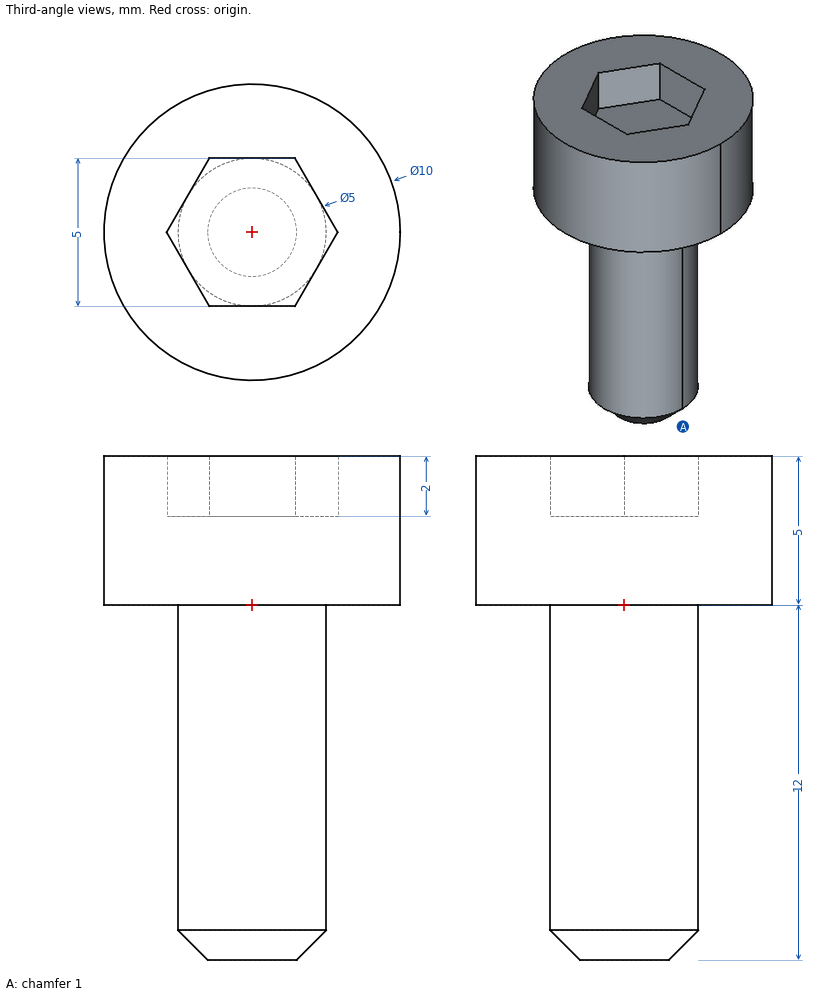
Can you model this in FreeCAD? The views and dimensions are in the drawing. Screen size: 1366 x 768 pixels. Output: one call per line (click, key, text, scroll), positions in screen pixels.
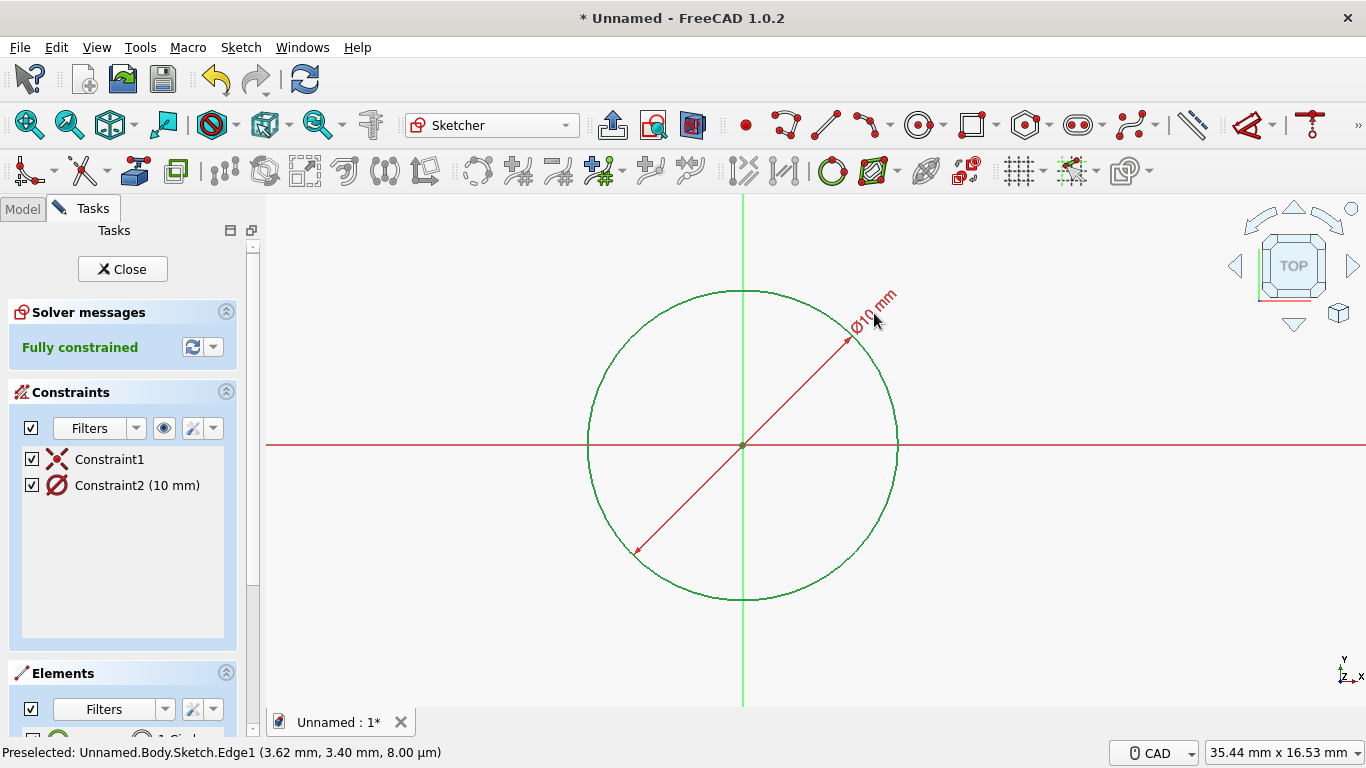
click(123, 269)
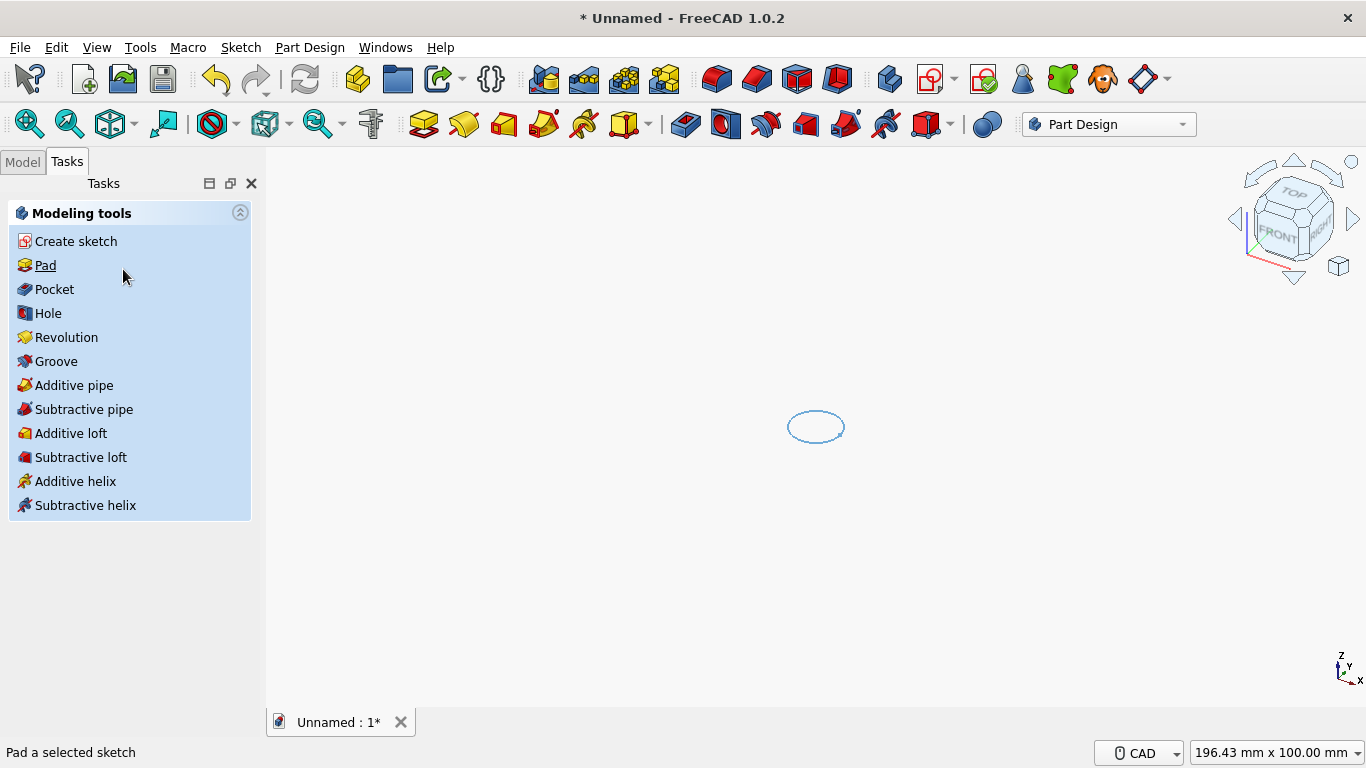
click(424, 124)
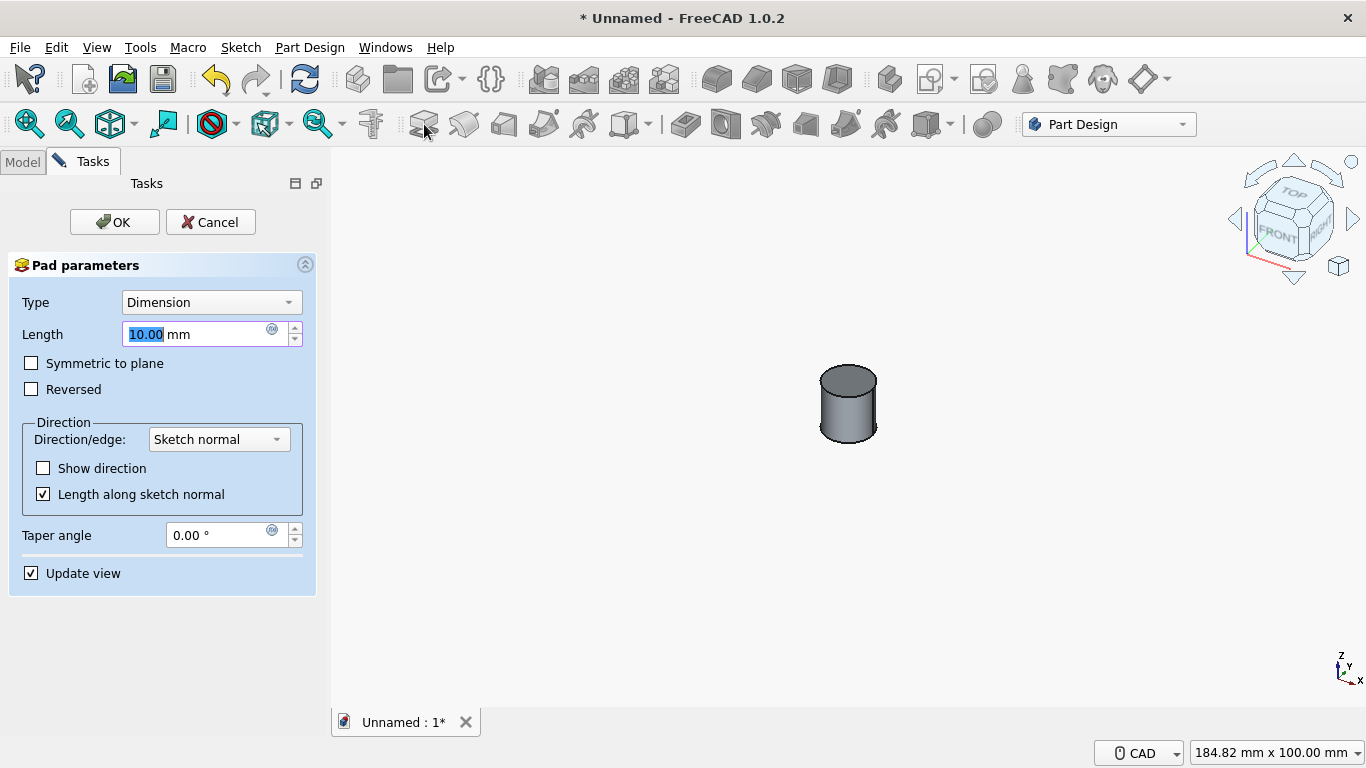
text(5)
key(Tab)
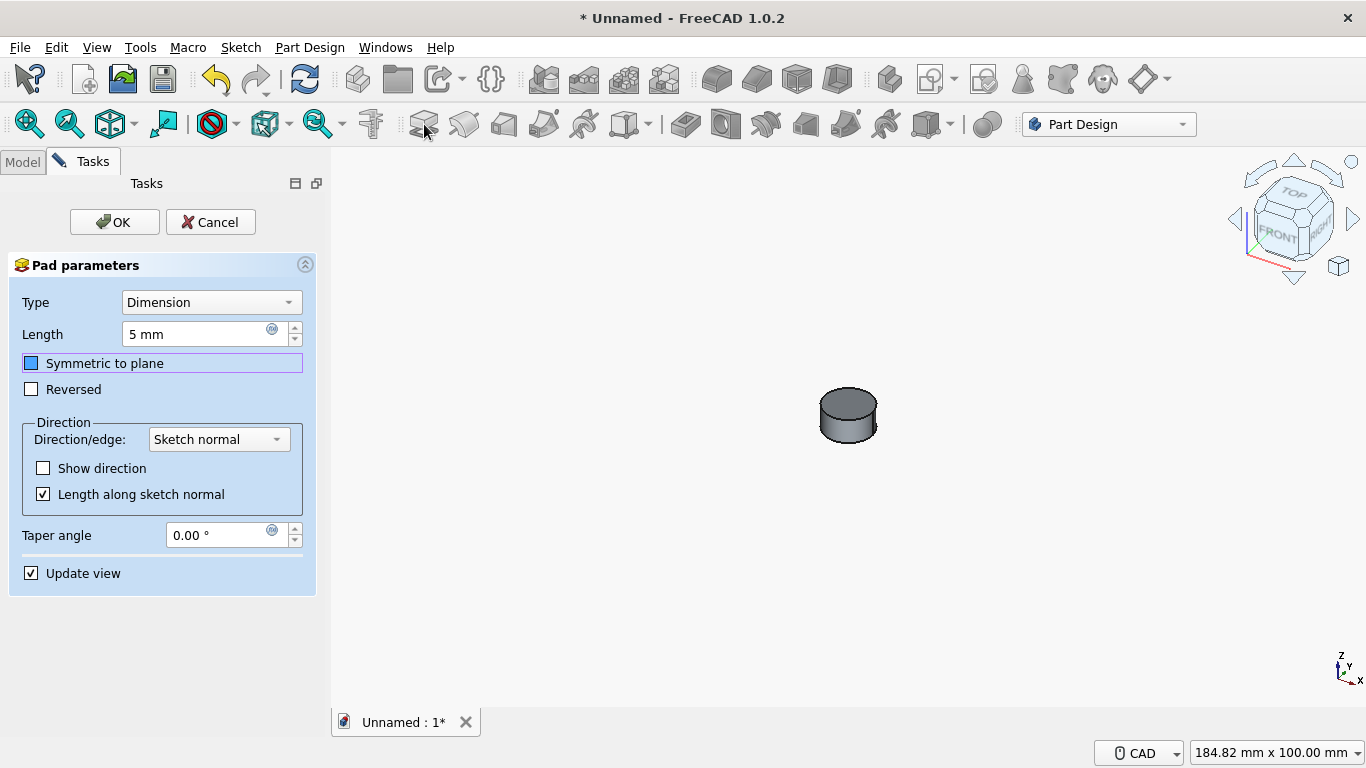
click(115, 222)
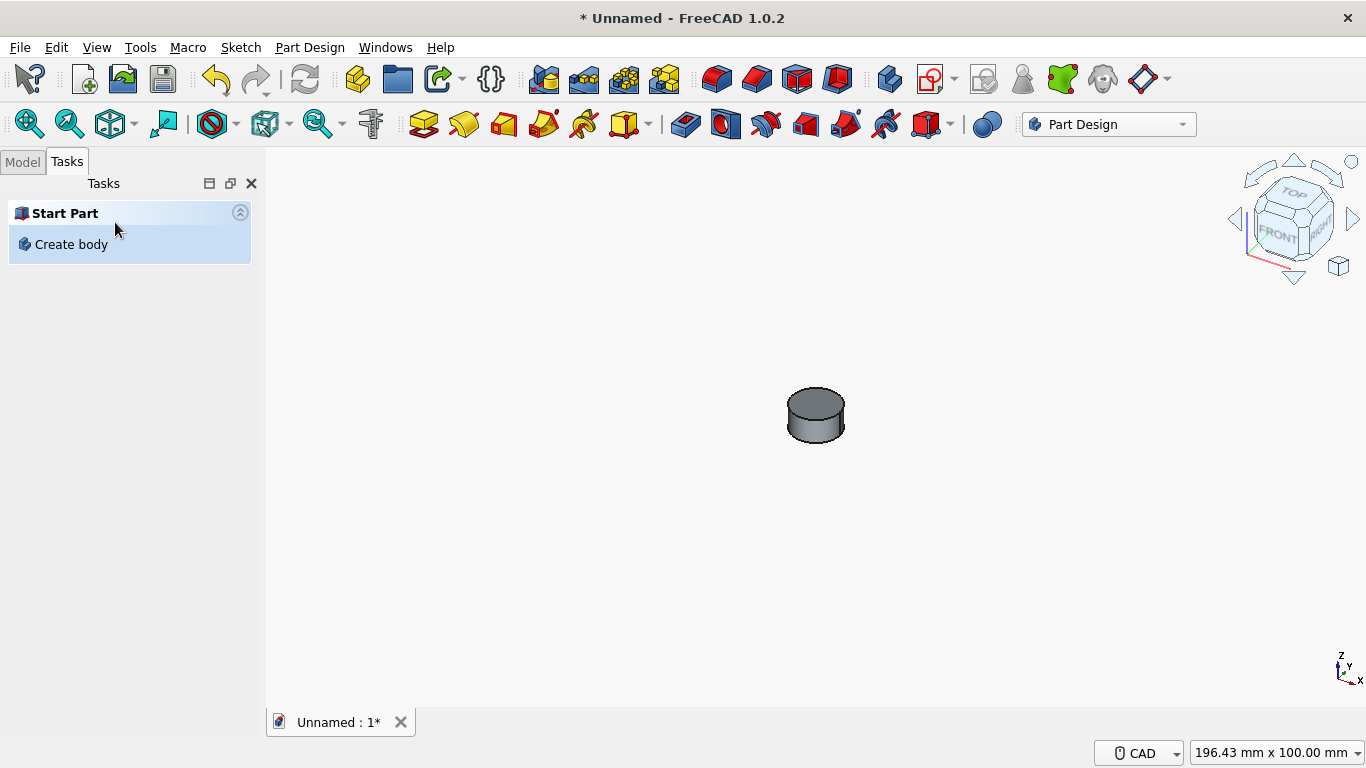
click(30, 124)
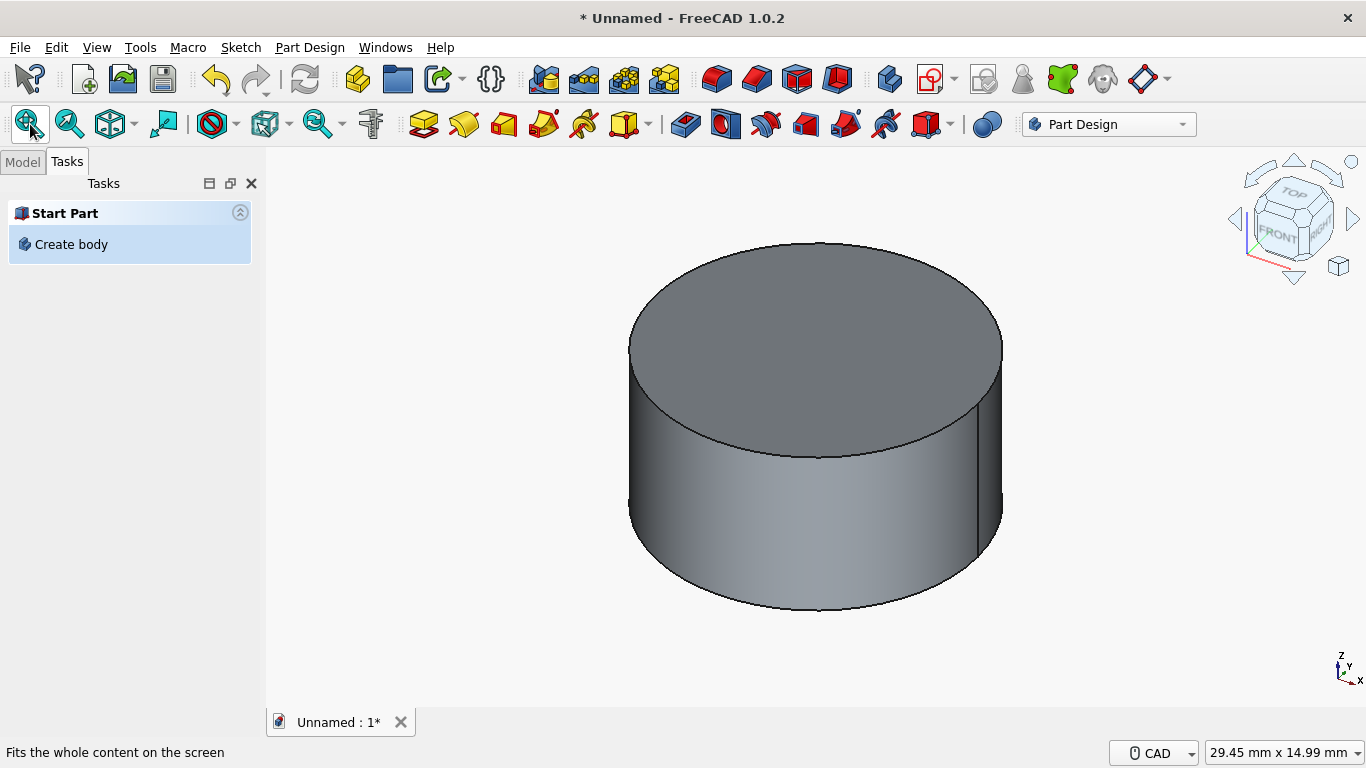
click(816, 349)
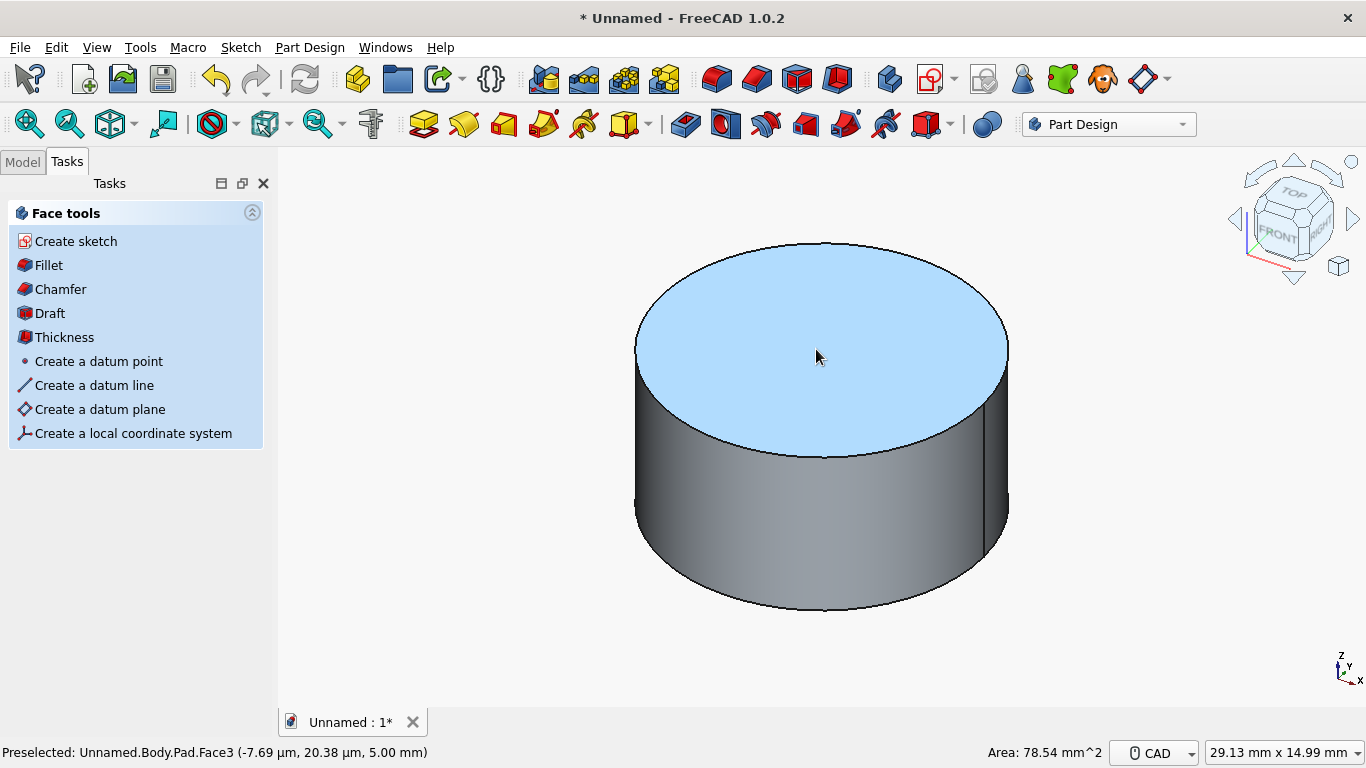
click(930, 80)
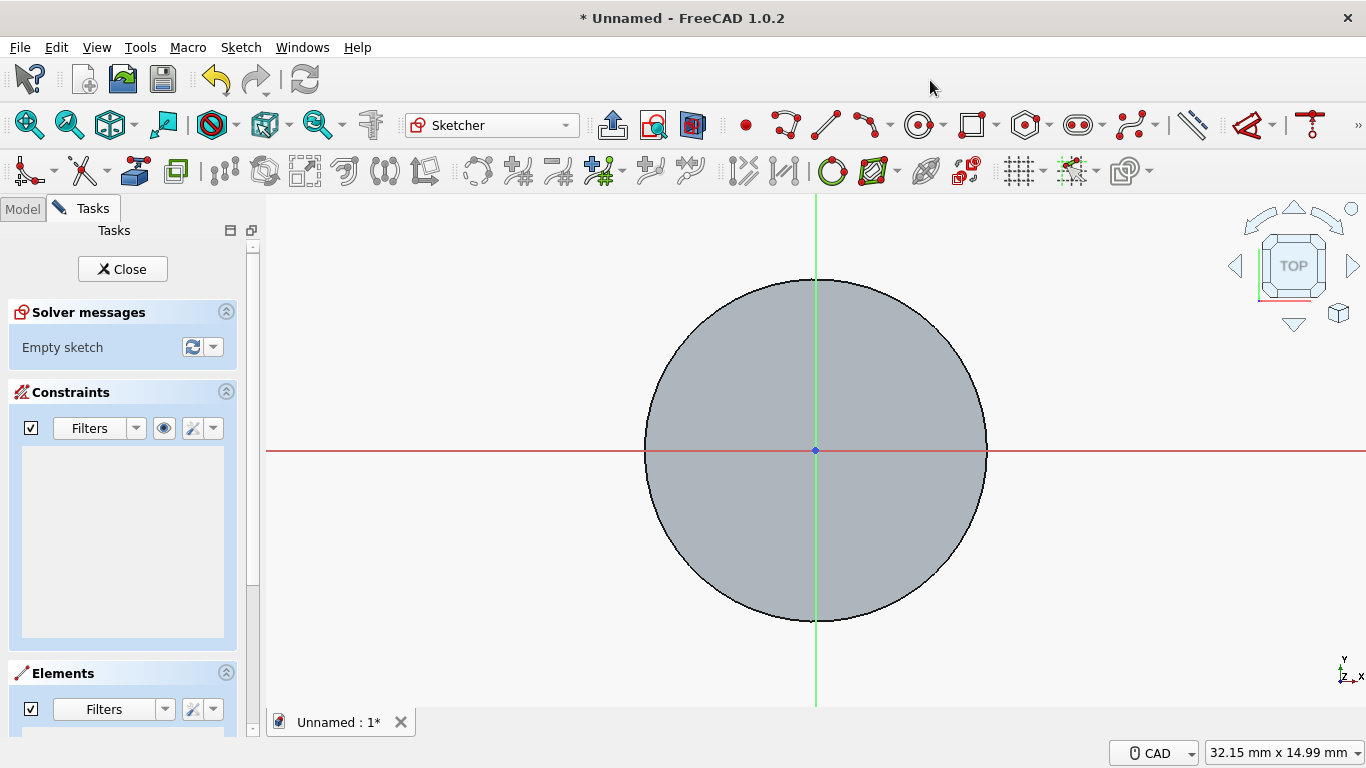
scroll(899, 450, up, 3)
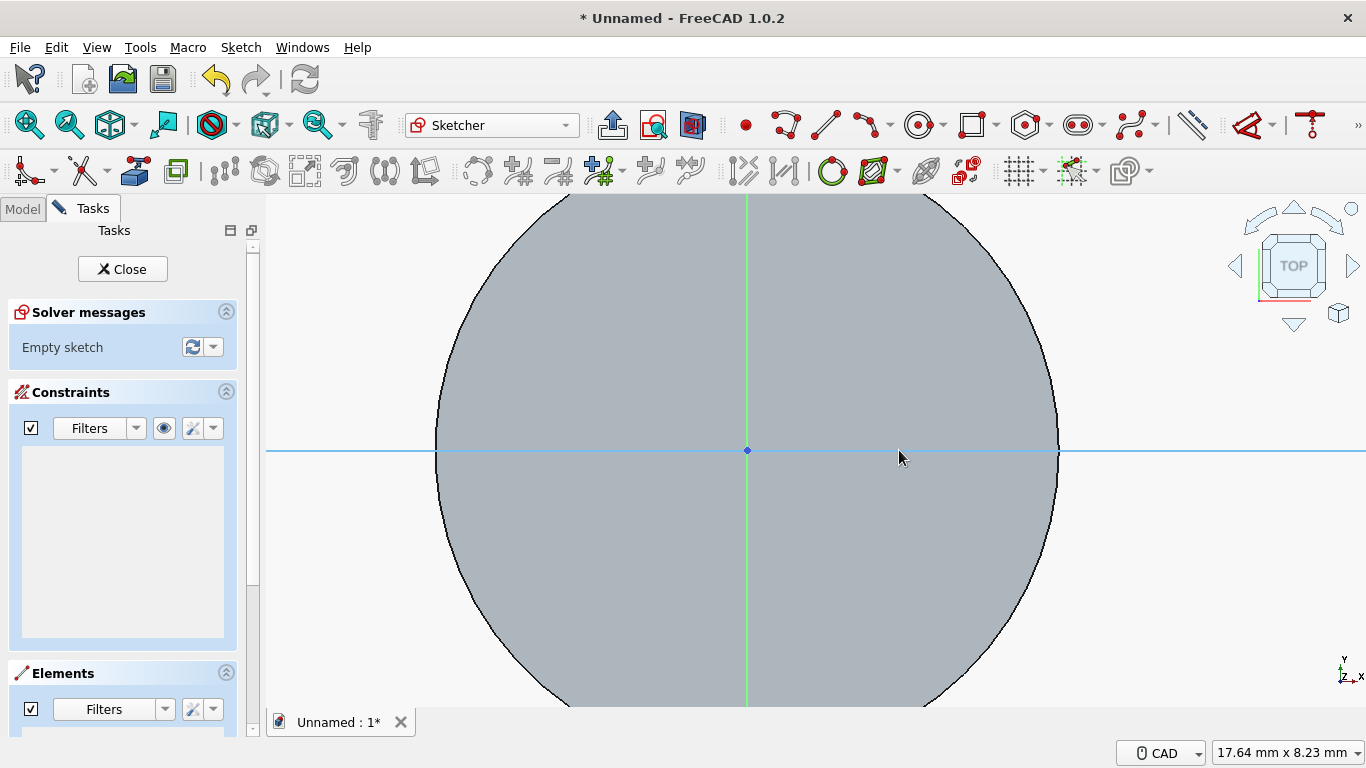
click(1026, 126)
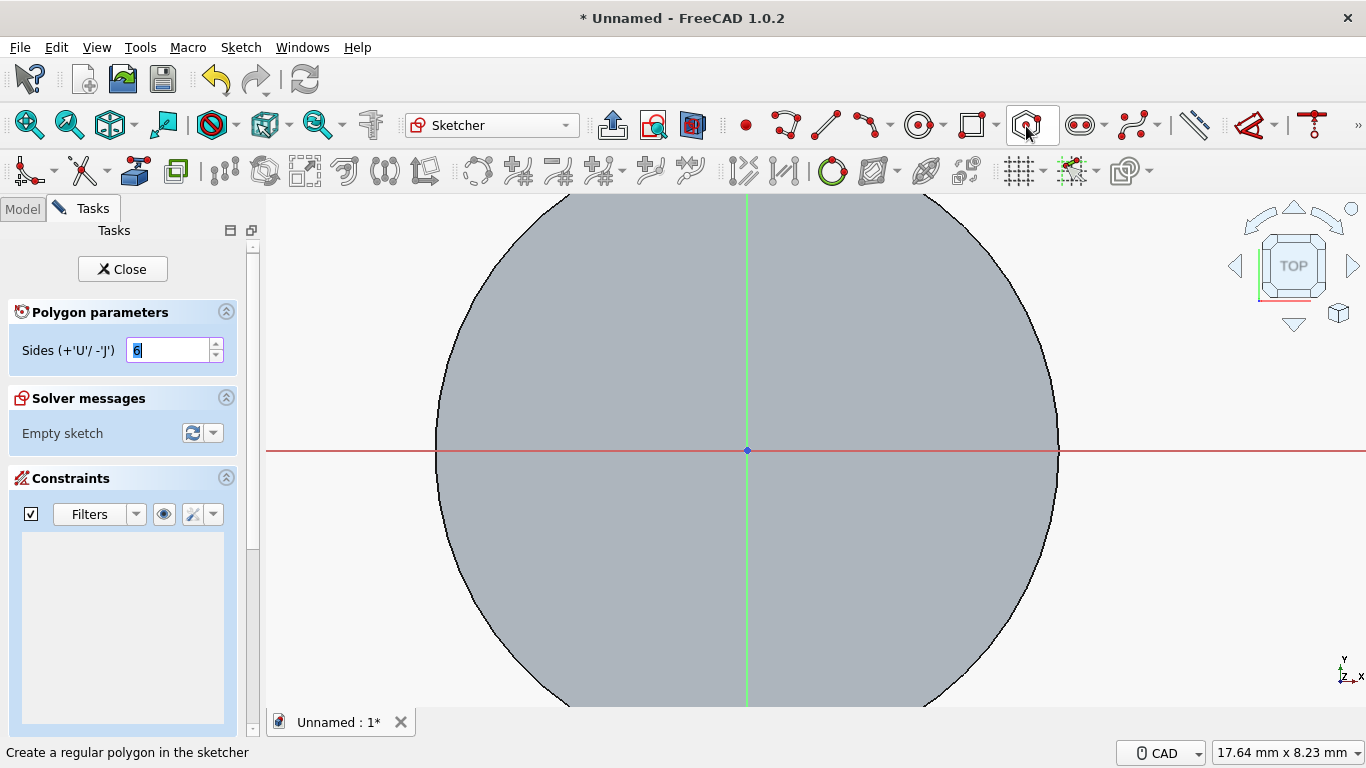
click(747, 450)